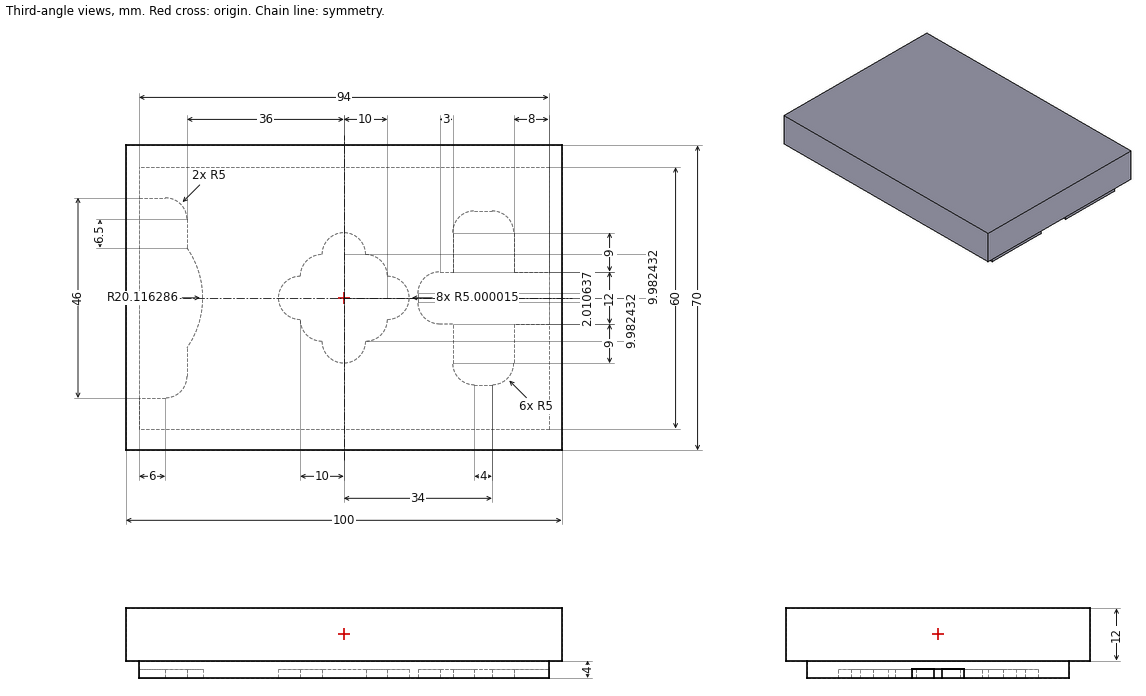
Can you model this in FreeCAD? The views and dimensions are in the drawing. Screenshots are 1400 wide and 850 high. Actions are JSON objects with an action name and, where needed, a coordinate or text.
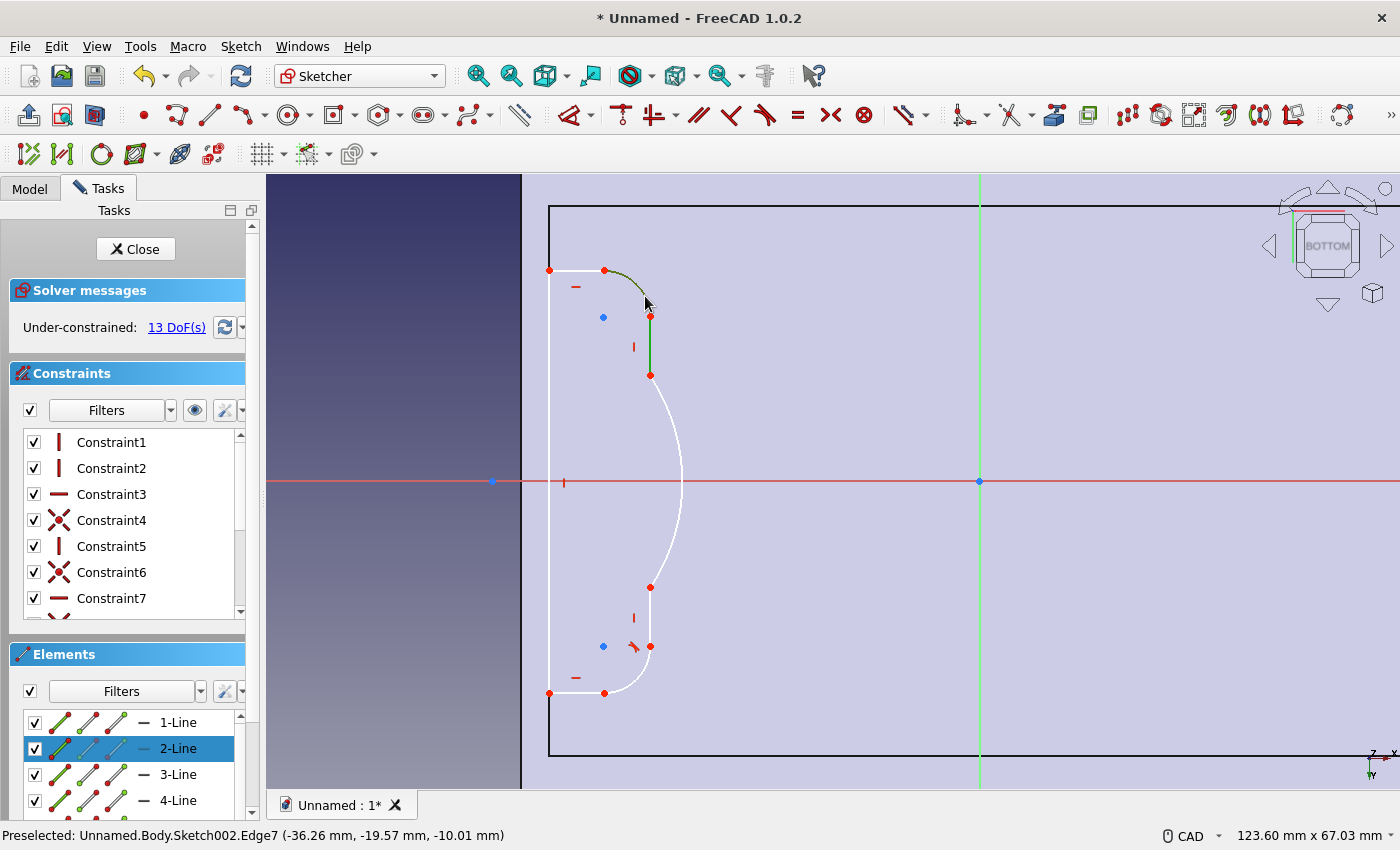
{"action": "left_click", "coordinate": [765, 116]}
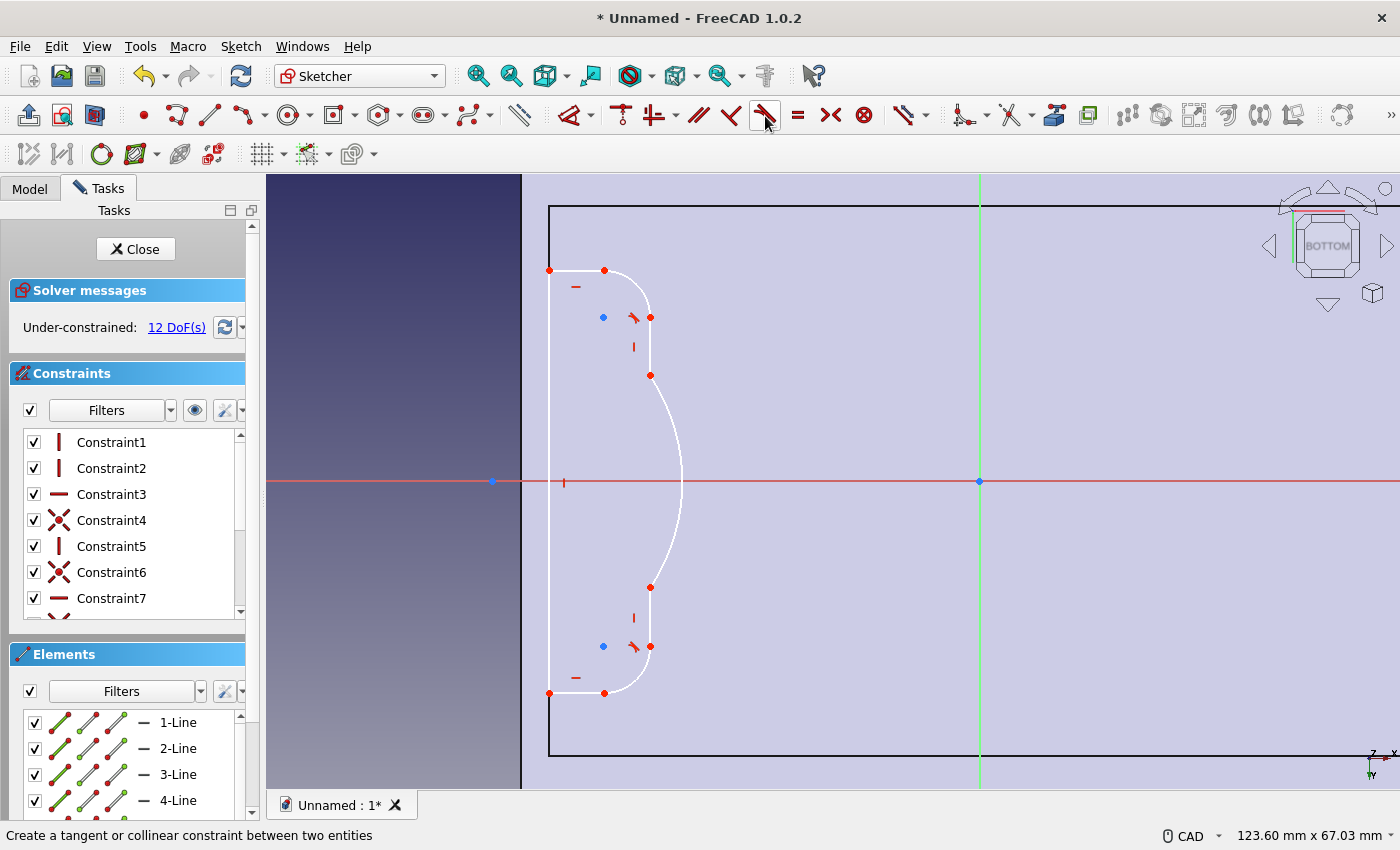
{"action": "left_click", "coordinate": [588, 271]}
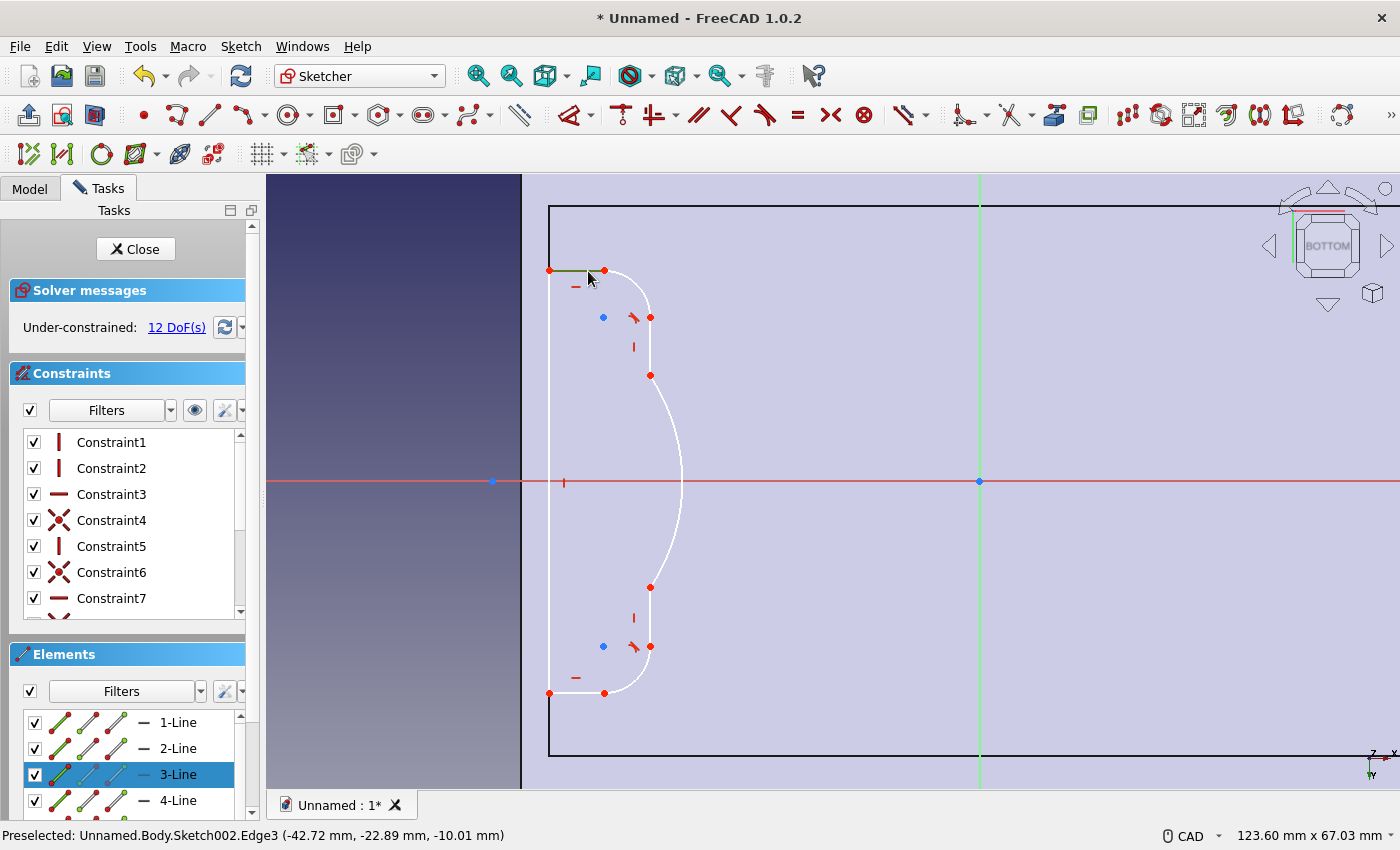
{"action": "left_click", "coordinate": [645, 296]}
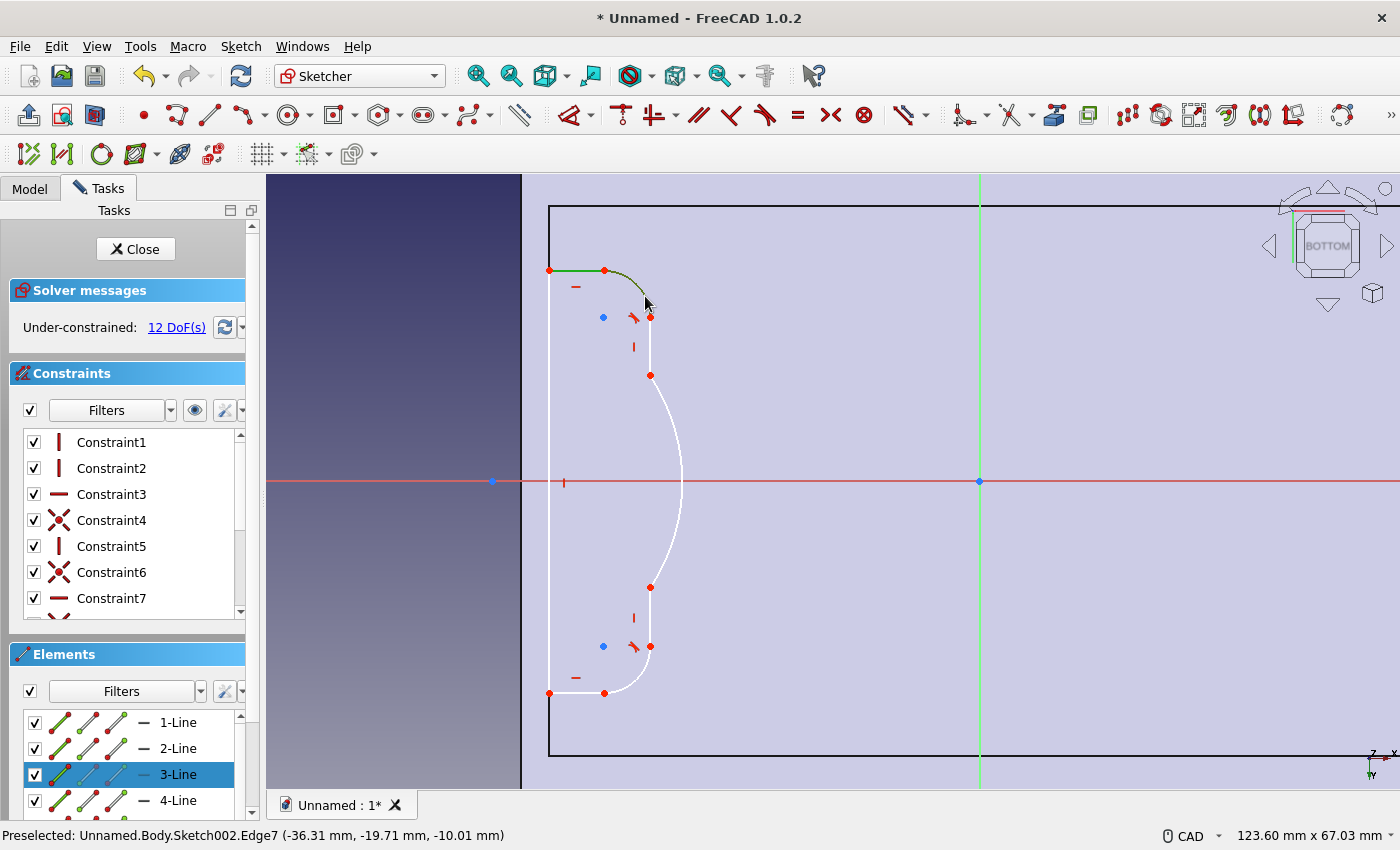
{"action": "left_click", "coordinate": [765, 116]}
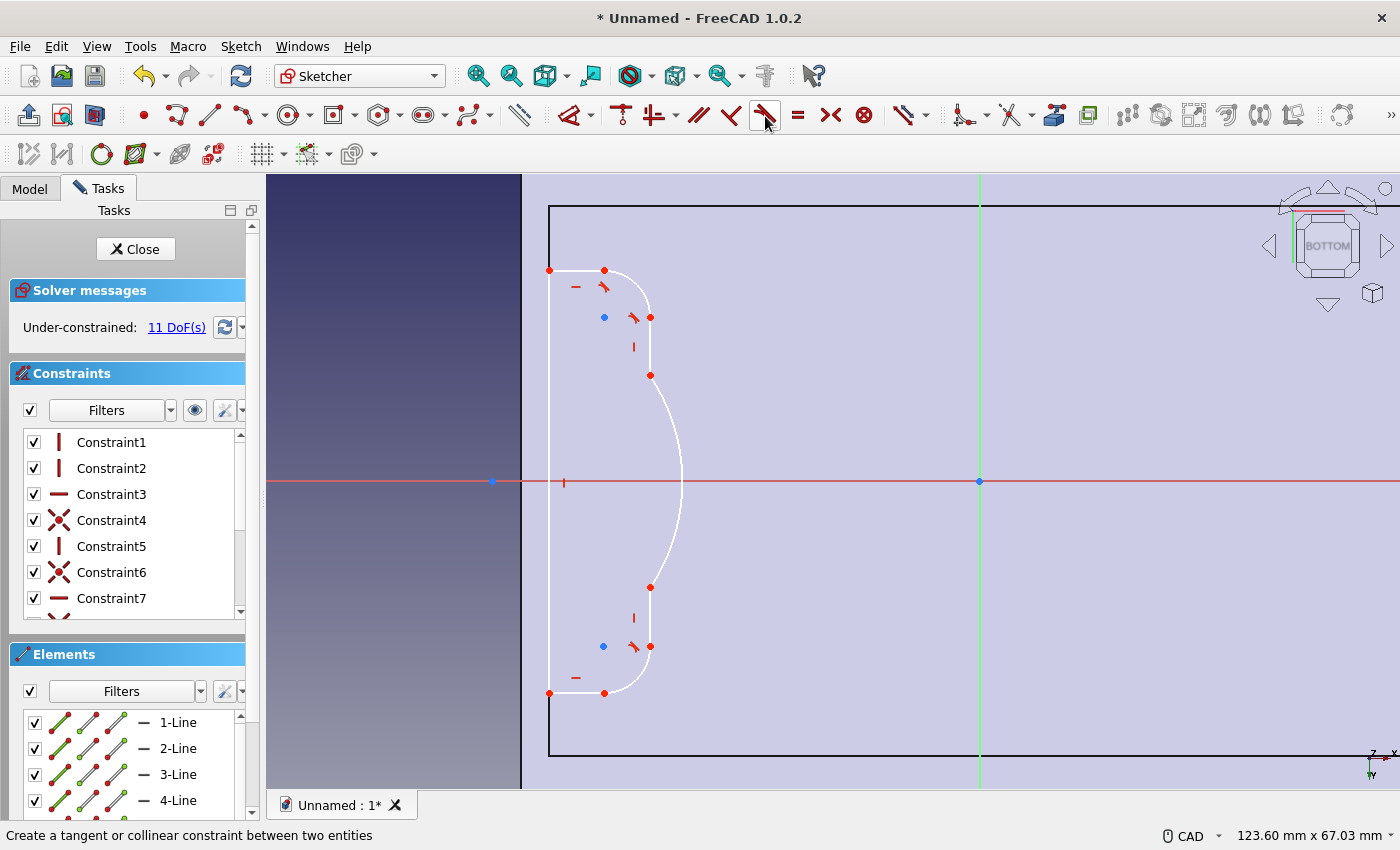
{"action": "left_click", "coordinate": [565, 693]}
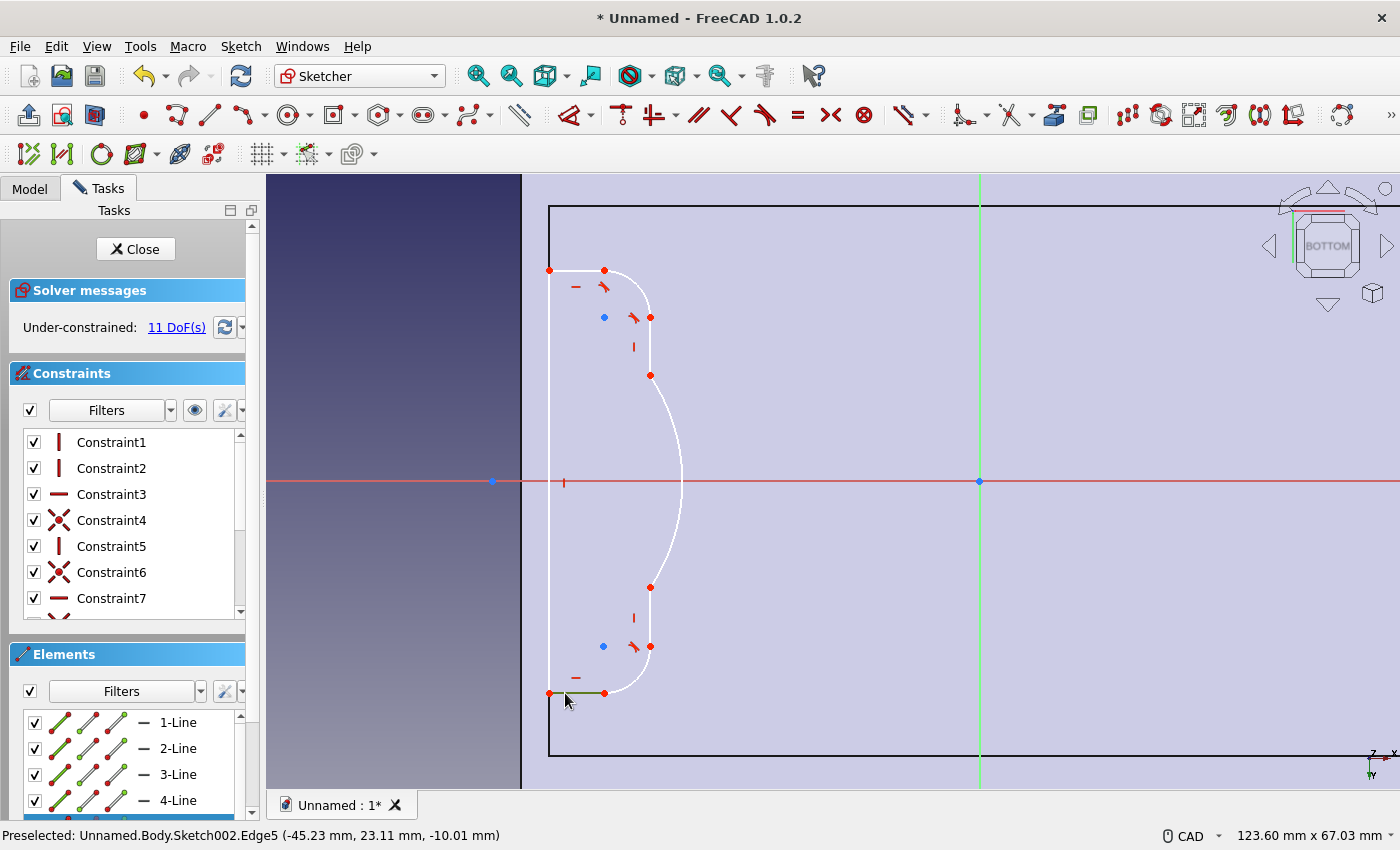
{"action": "left_click", "coordinate": [625, 688]}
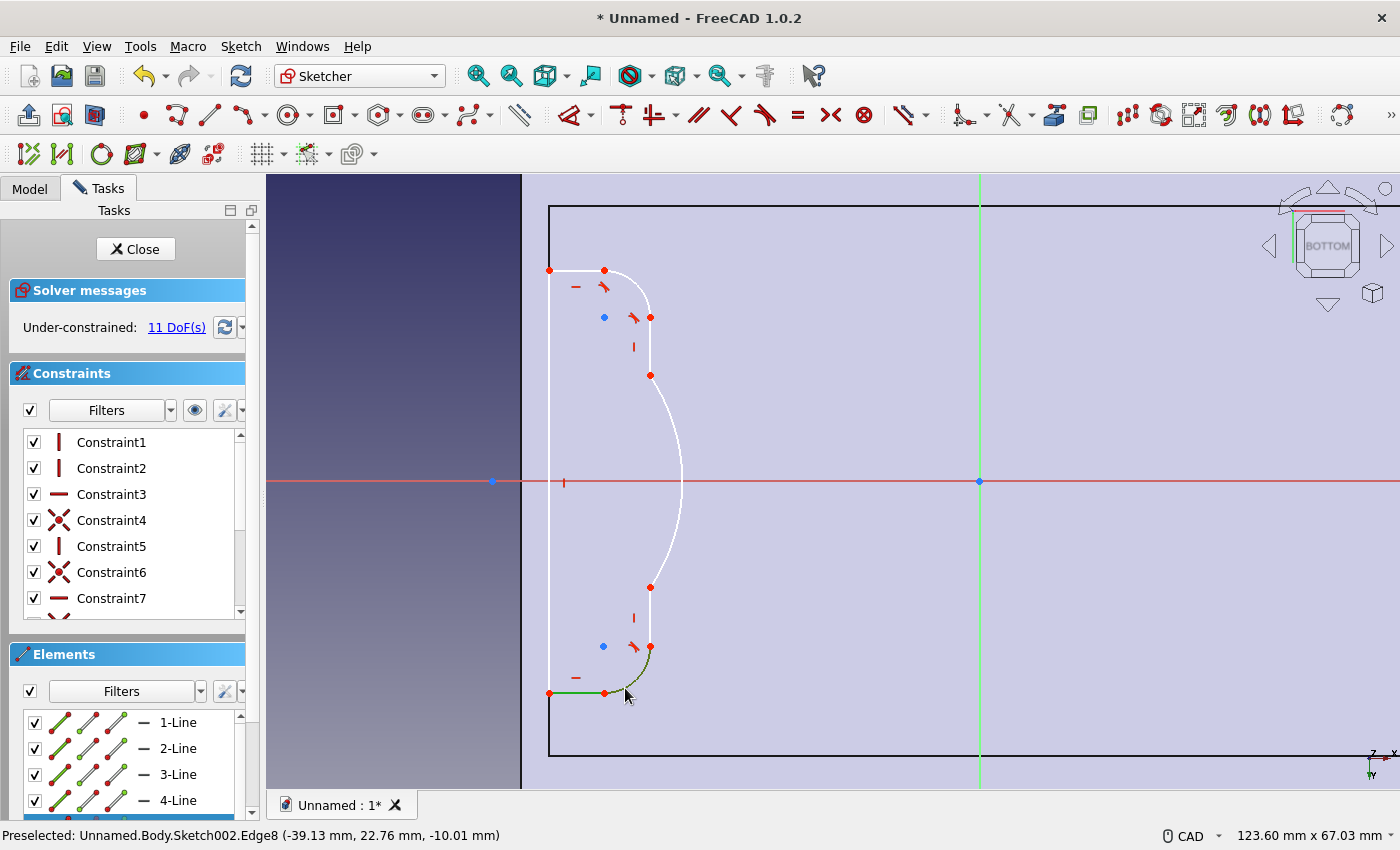
{"action": "left_click", "coordinate": [765, 116]}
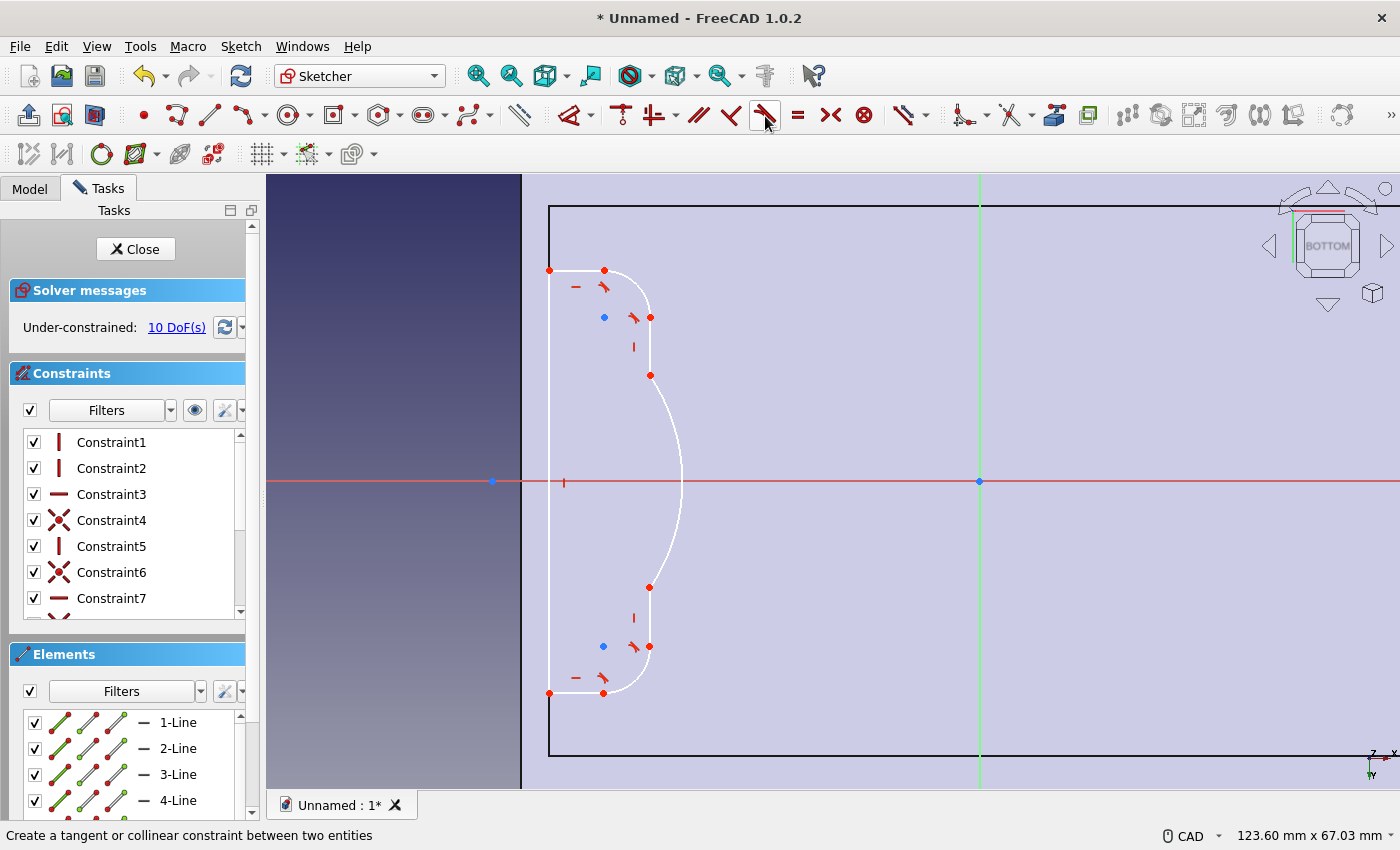
{"action": "left_click", "coordinate": [645, 296]}